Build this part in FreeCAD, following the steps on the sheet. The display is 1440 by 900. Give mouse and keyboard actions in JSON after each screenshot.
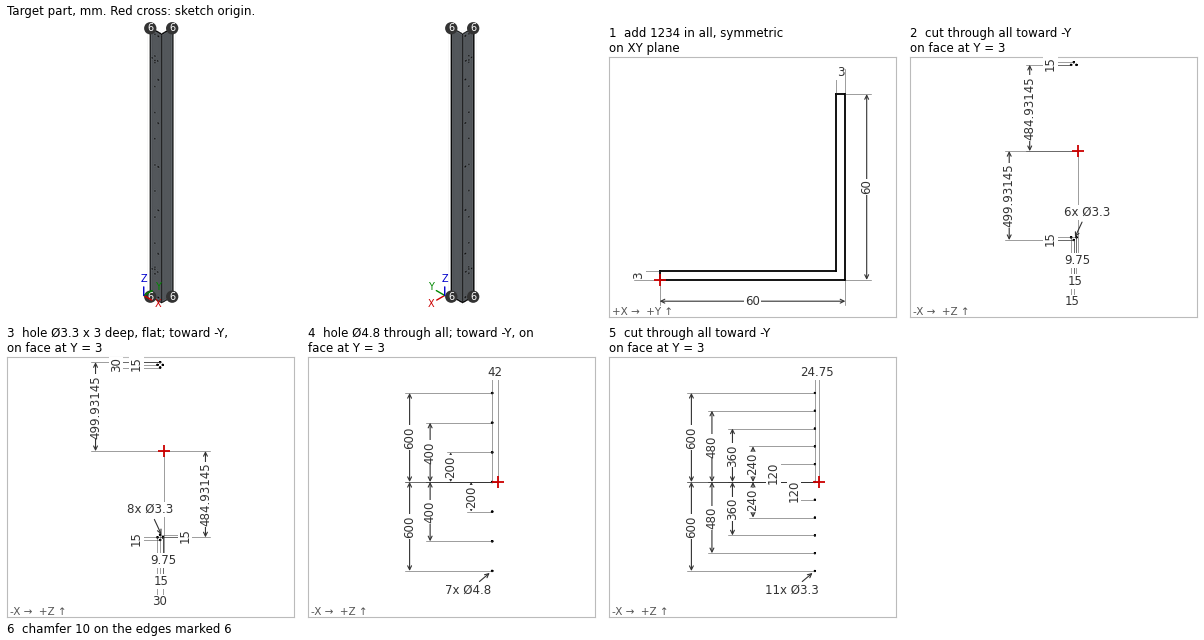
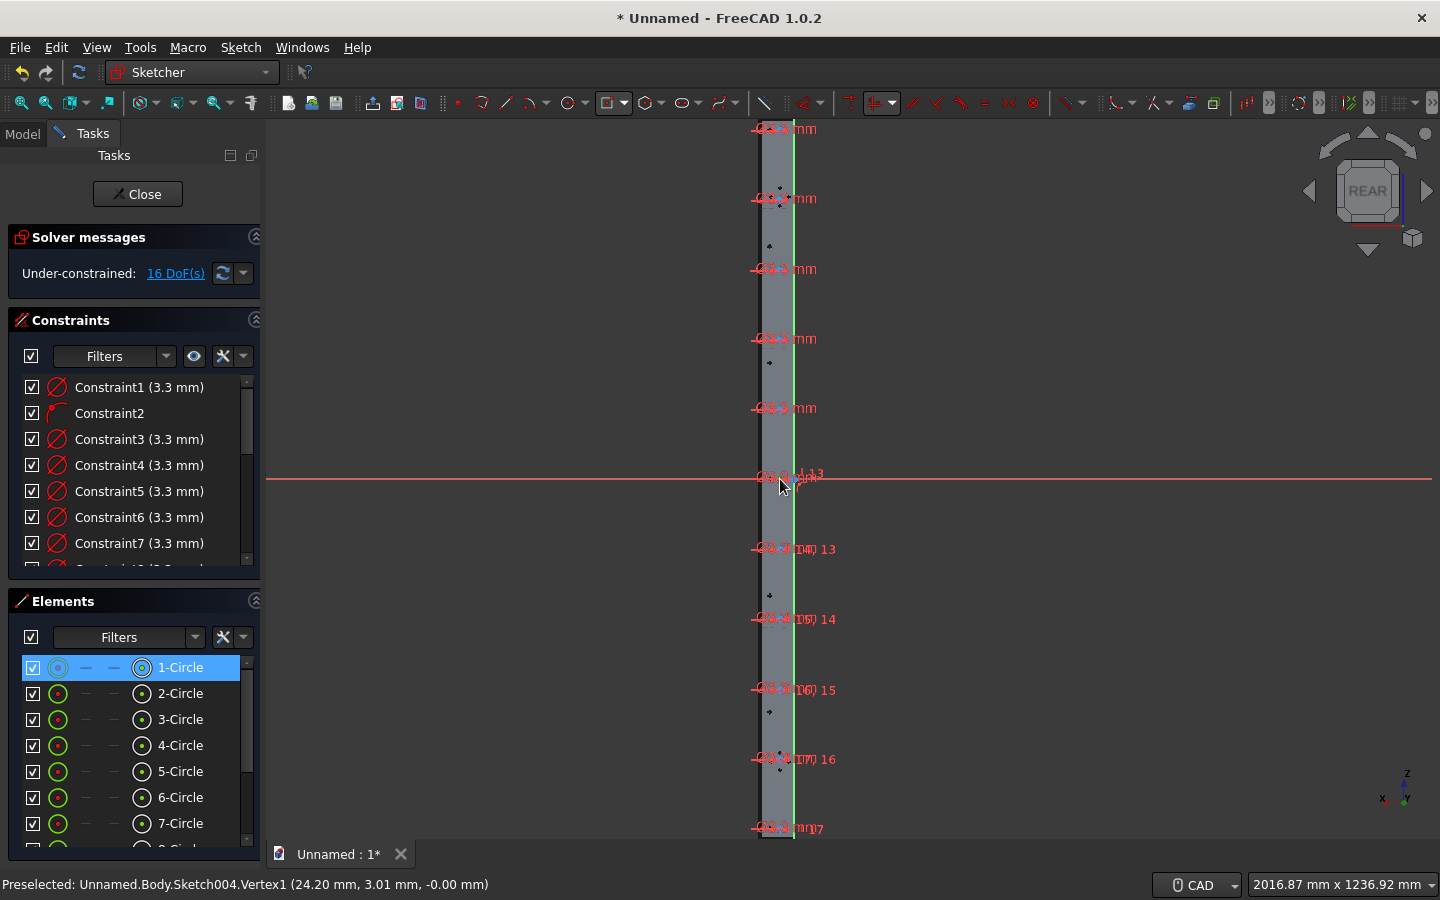
{"action": "scroll", "coordinate": [780, 478], "scroll_direction": "down", "scroll_amount": 2}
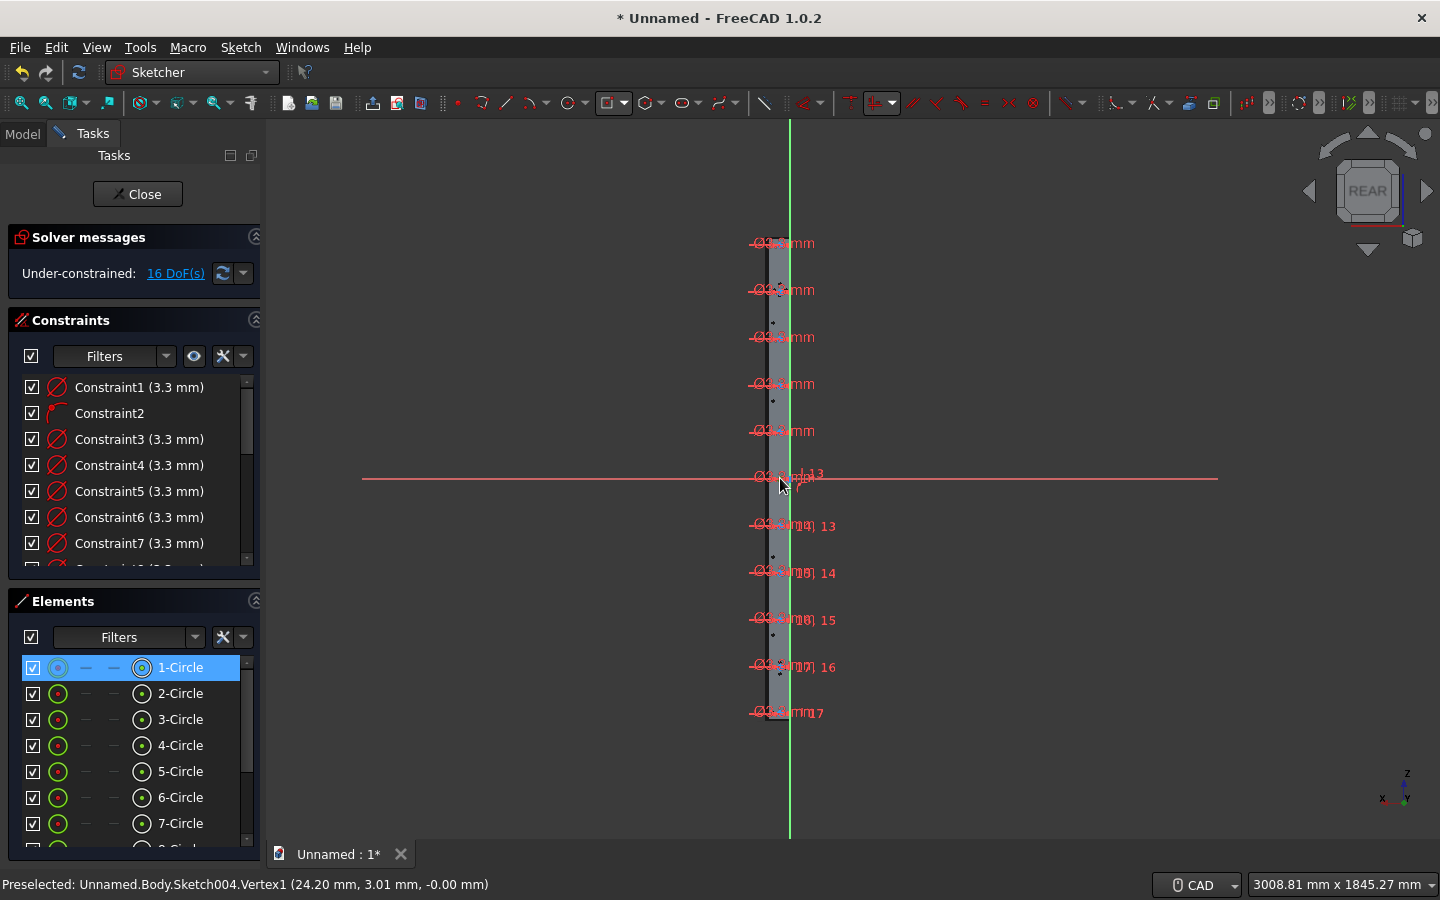
{"action": "left_click", "coordinate": [780, 245]}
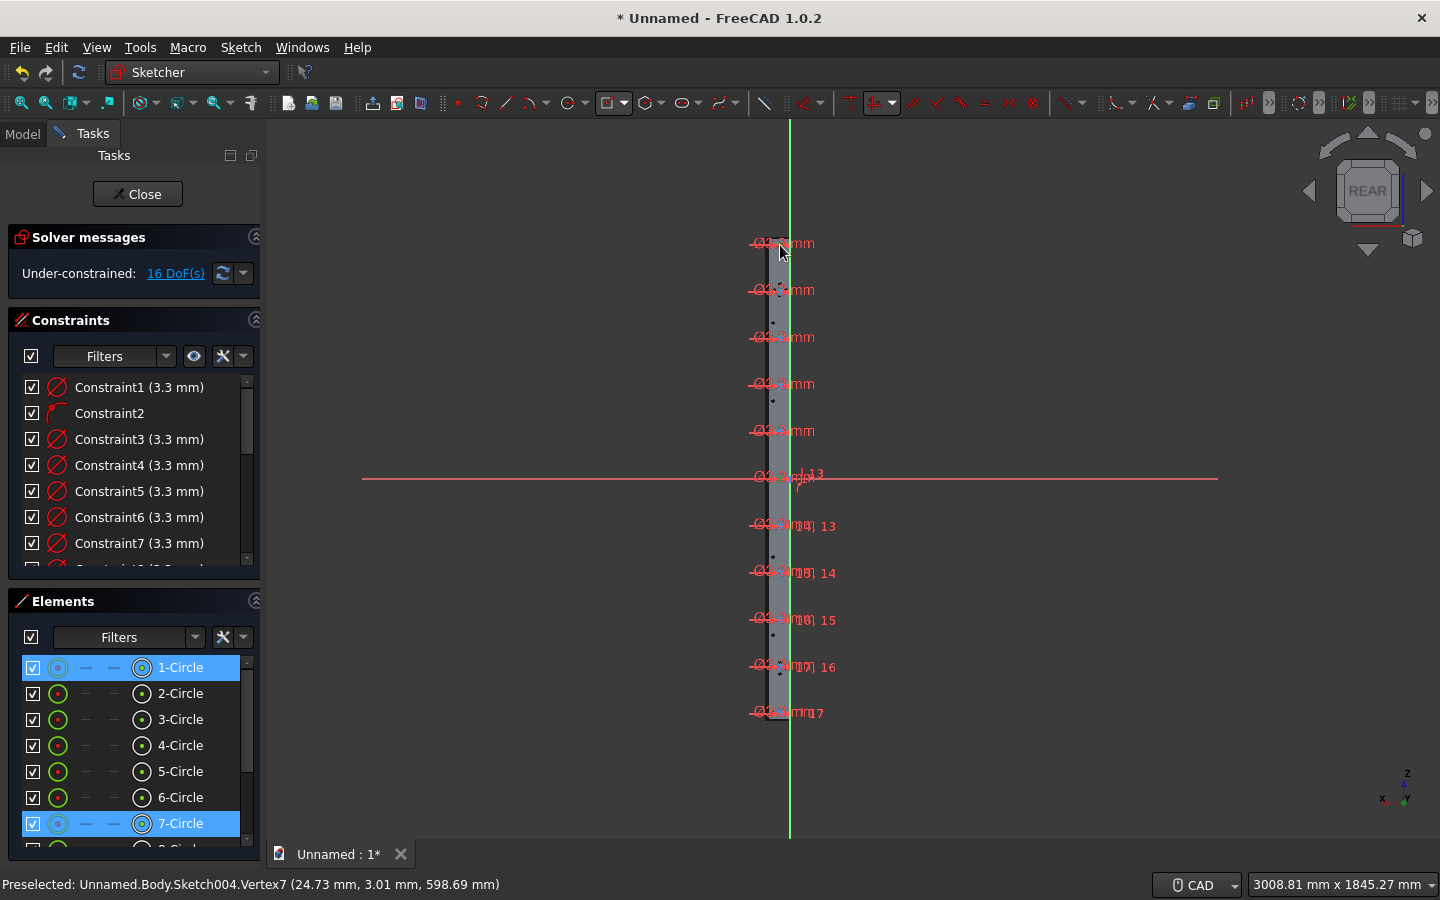
{"action": "left_click", "coordinate": [894, 104]}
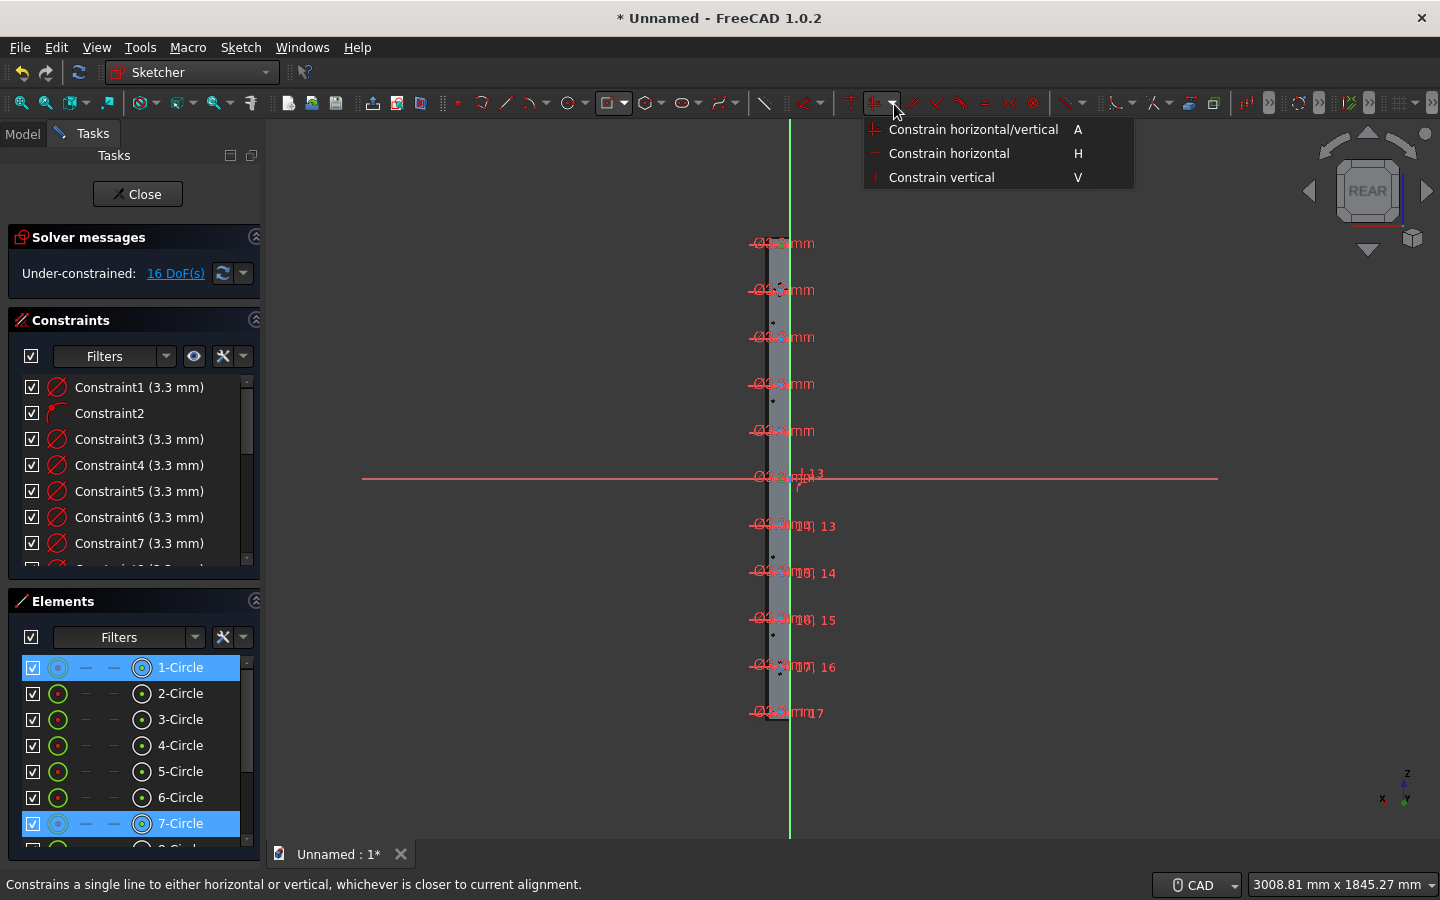
{"action": "left_click", "coordinate": [999, 177]}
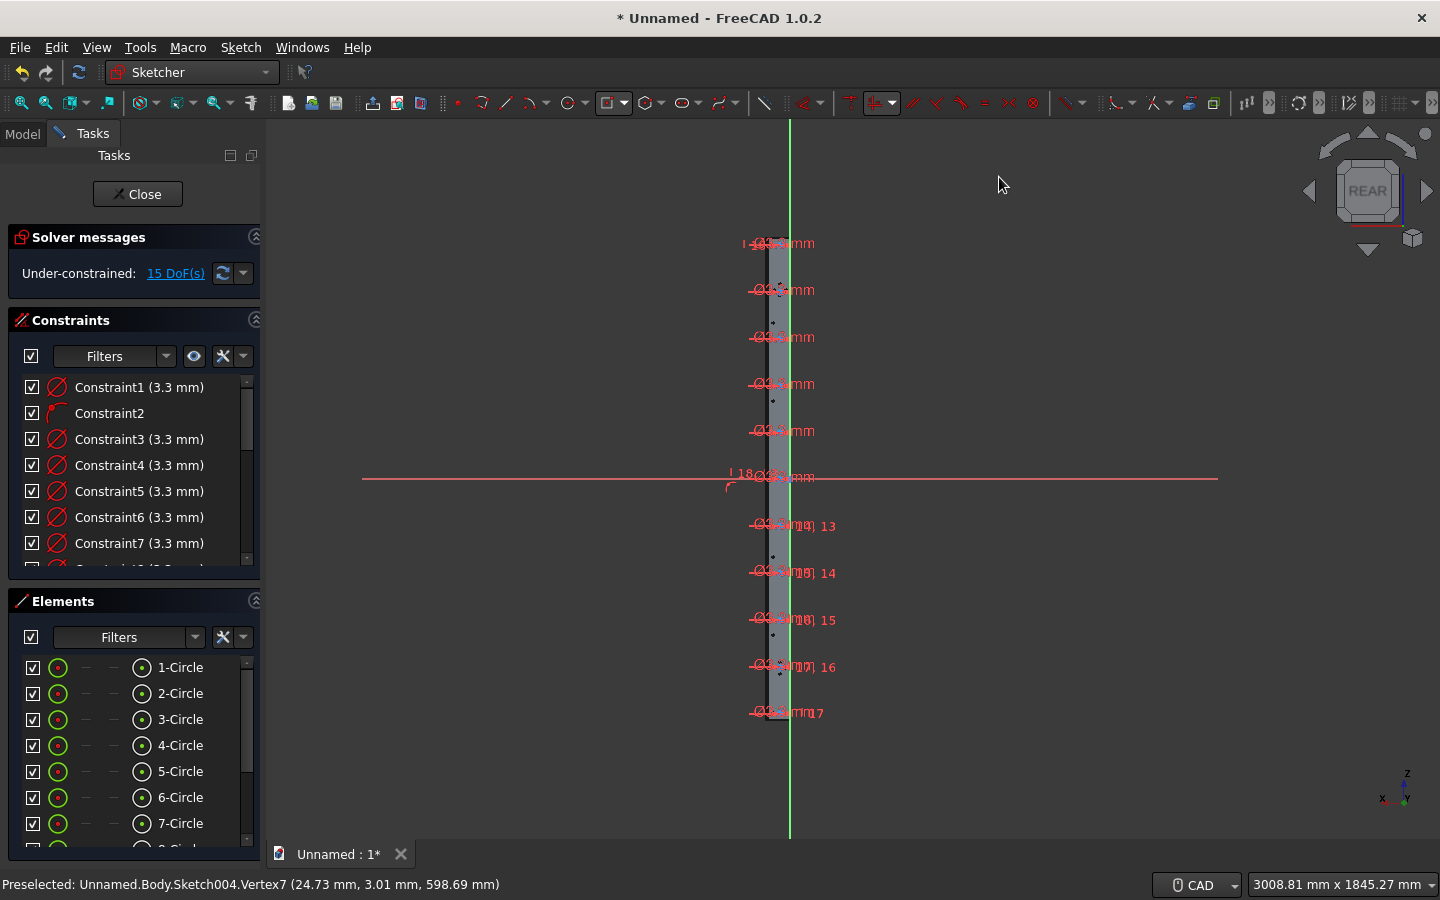
{"action": "left_click", "coordinate": [780, 245]}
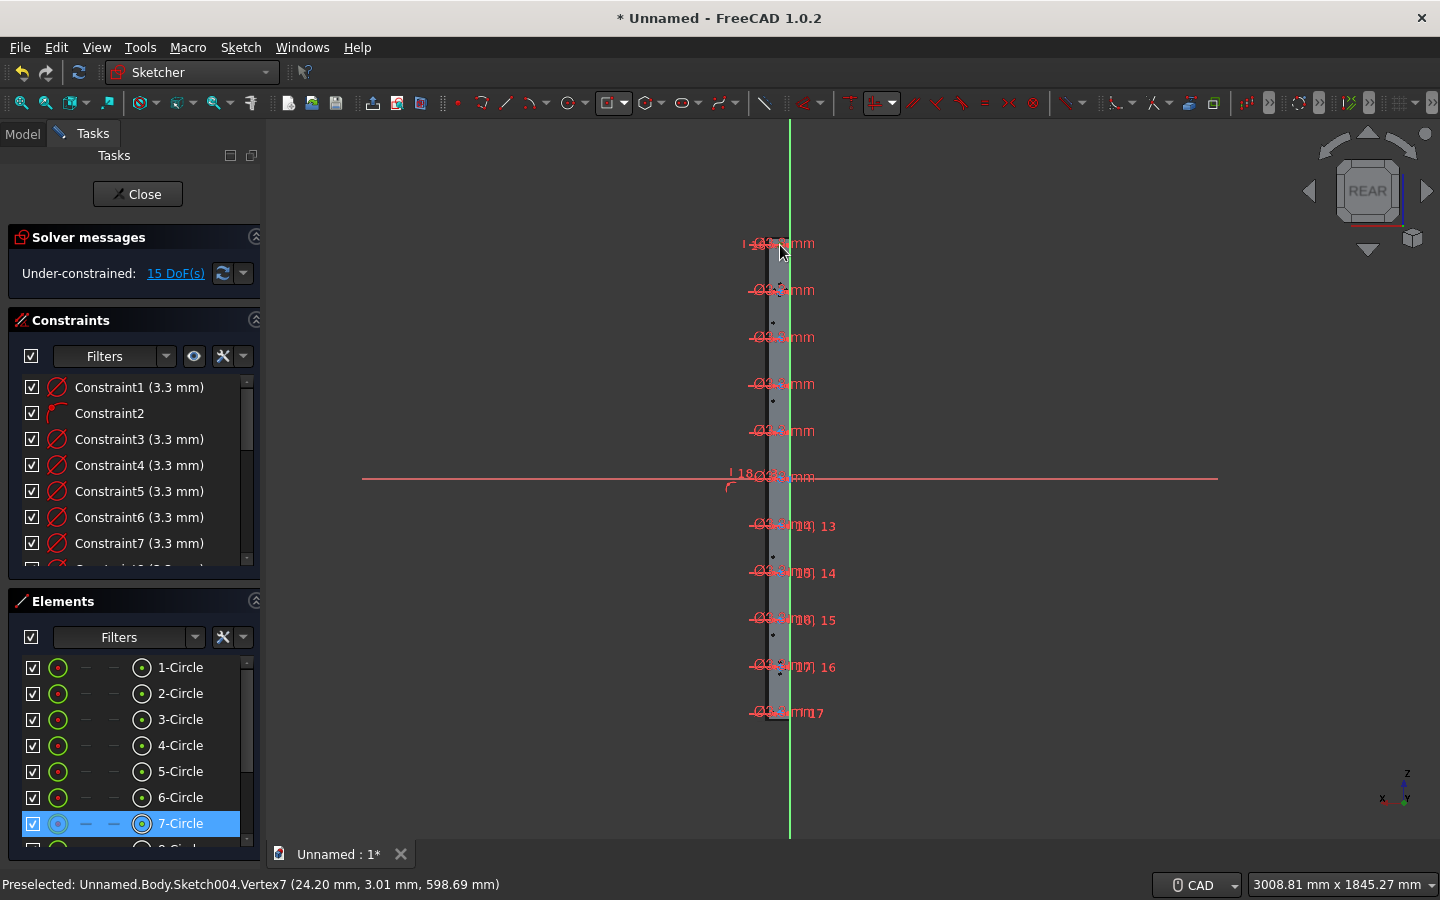
{"action": "left_click", "coordinate": [780, 292]}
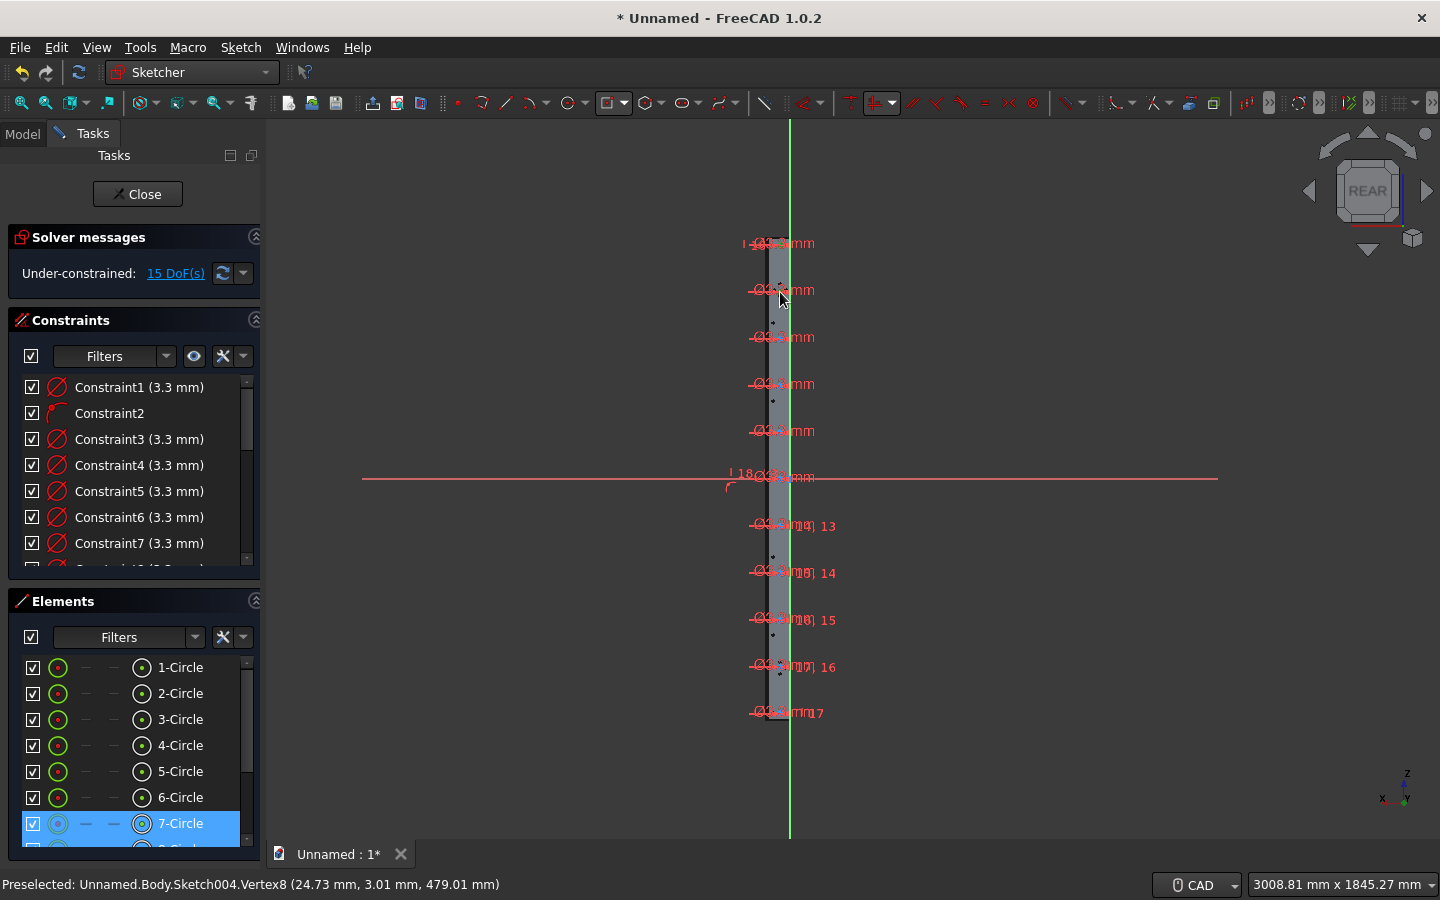
{"action": "key", "text": "v"}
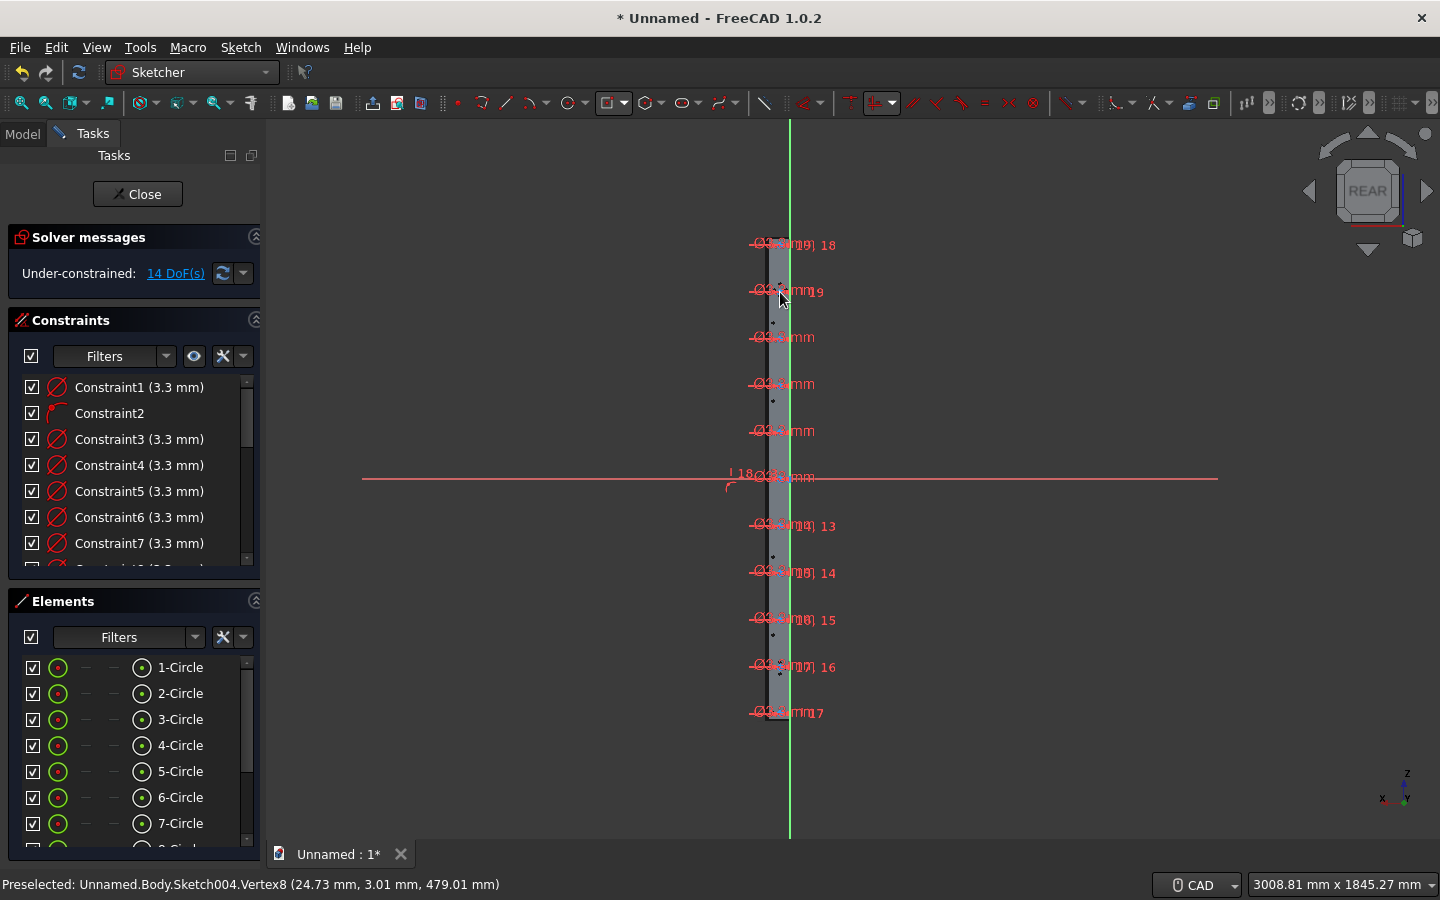
{"action": "left_click", "coordinate": [780, 292]}